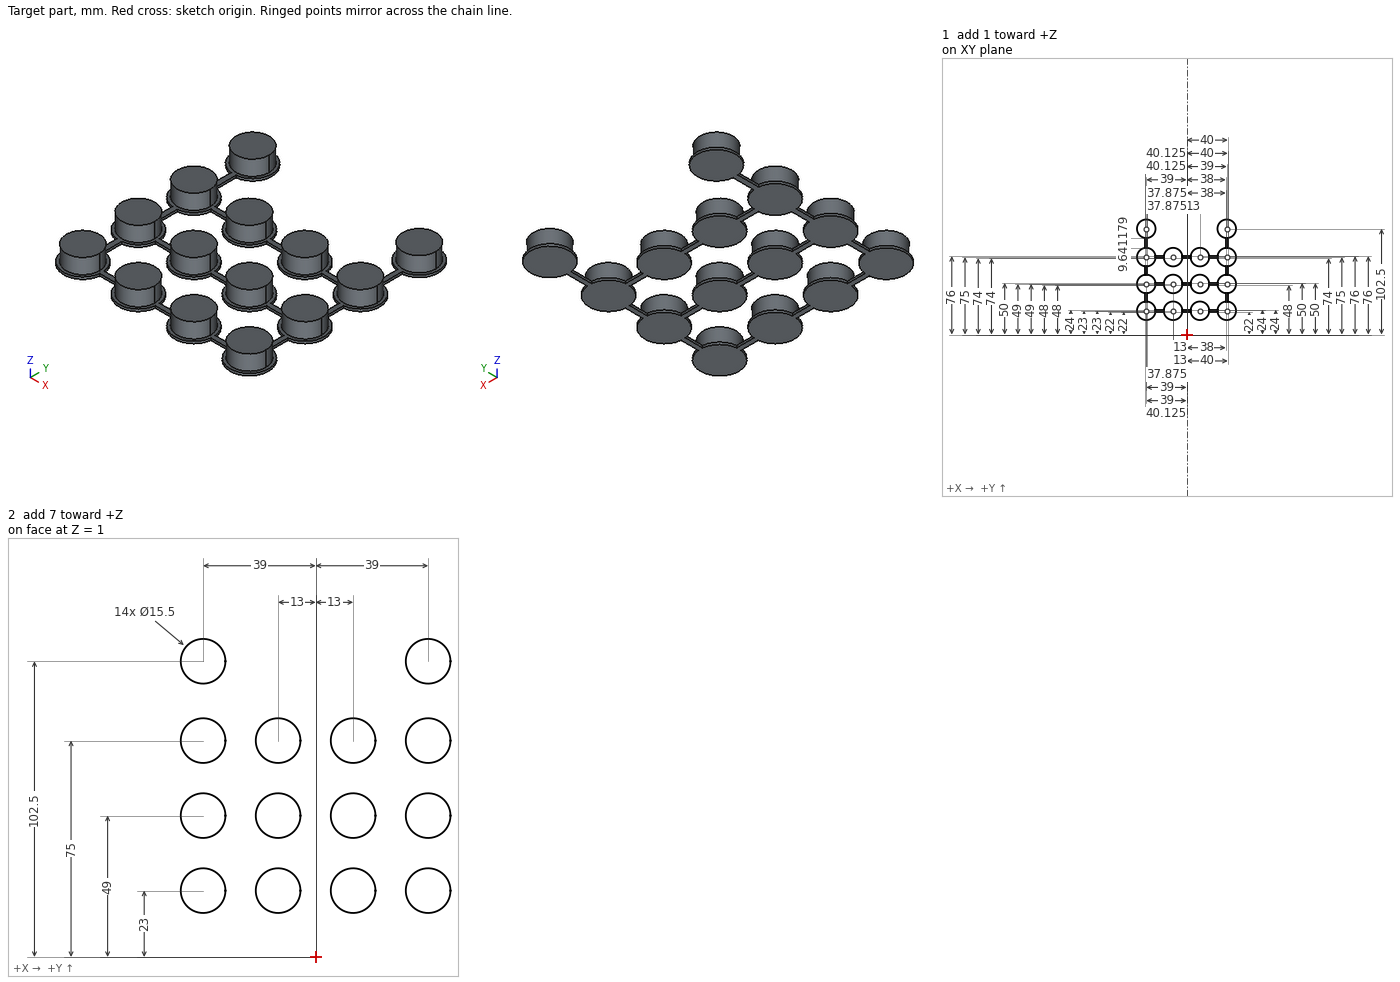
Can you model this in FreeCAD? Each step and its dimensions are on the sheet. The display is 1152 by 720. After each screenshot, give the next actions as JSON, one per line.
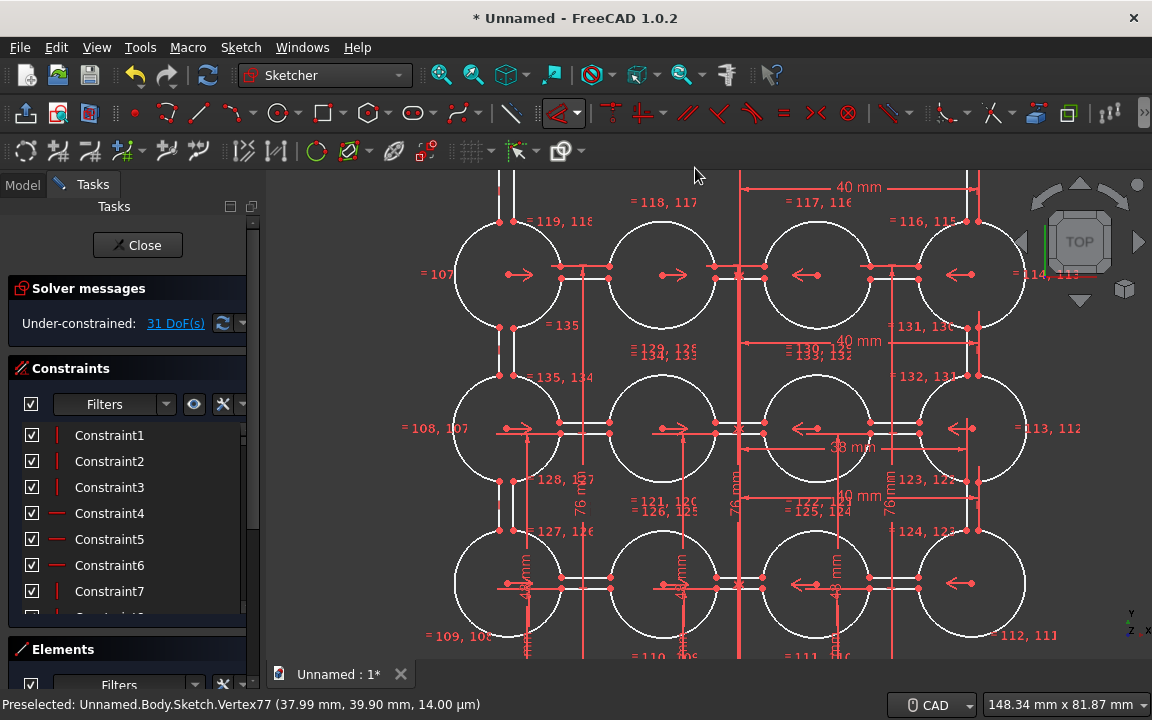
{"action": "left_click", "coordinate": [918, 578]}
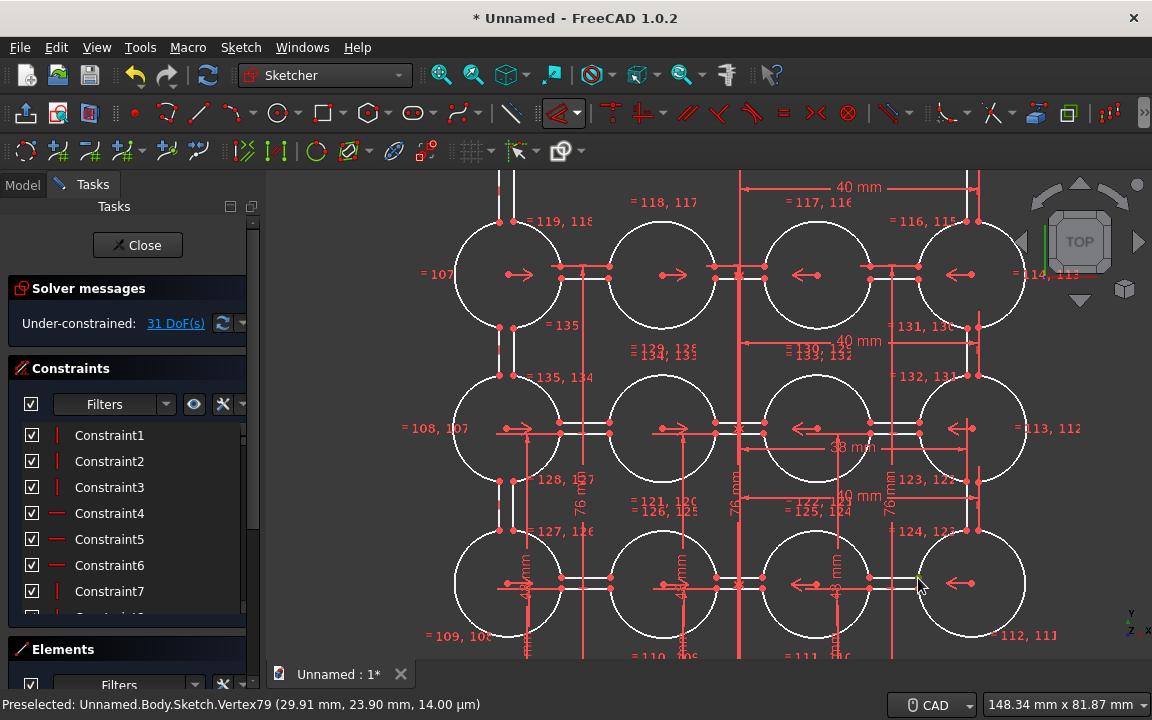
{"action": "key", "text": "i"}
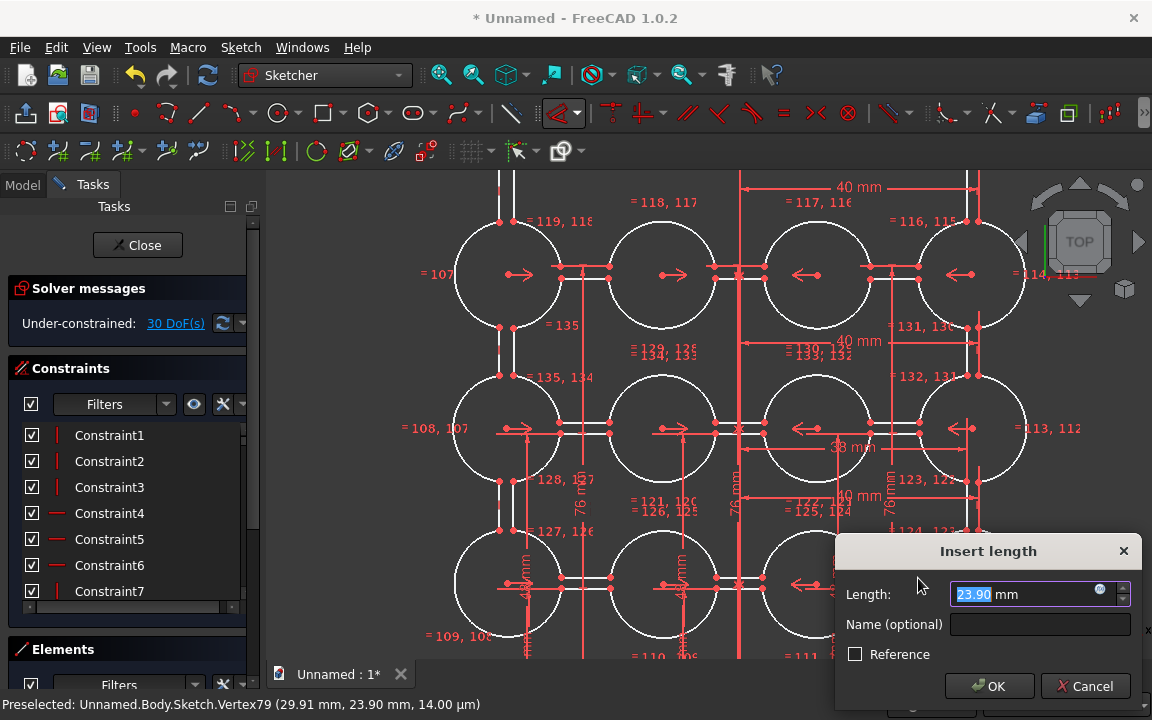
{"action": "type", "text": "24"}
{"action": "key", "text": "Return"}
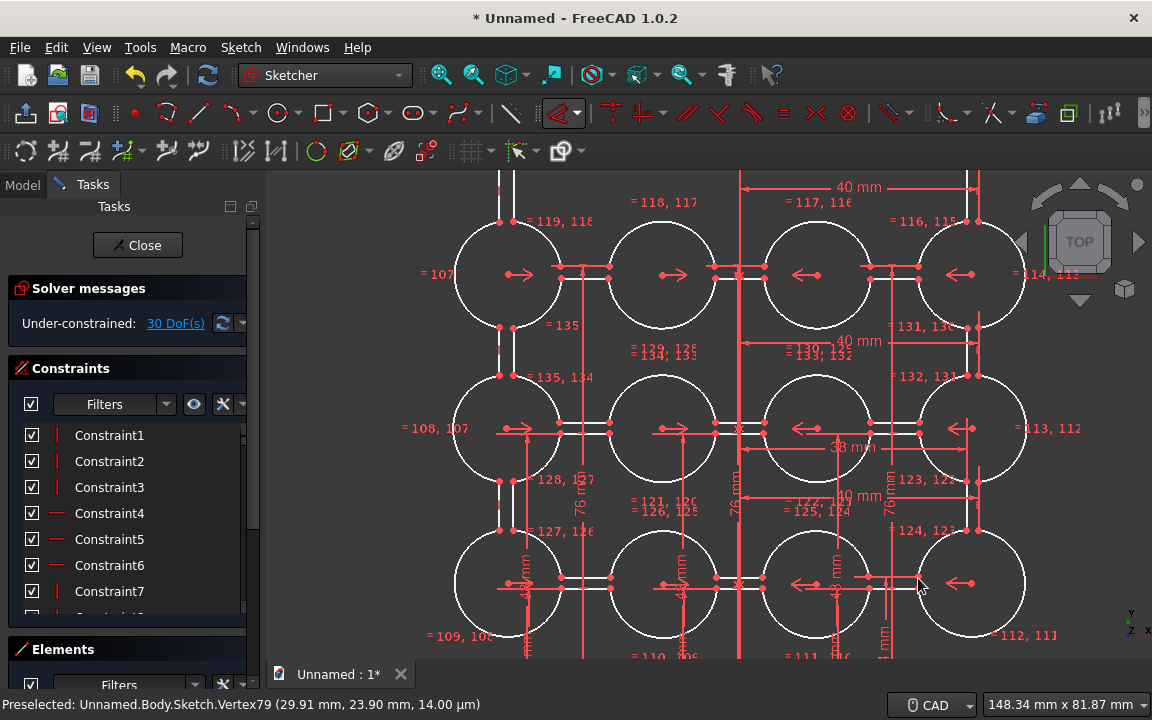
{"action": "left_click", "coordinate": [763, 578]}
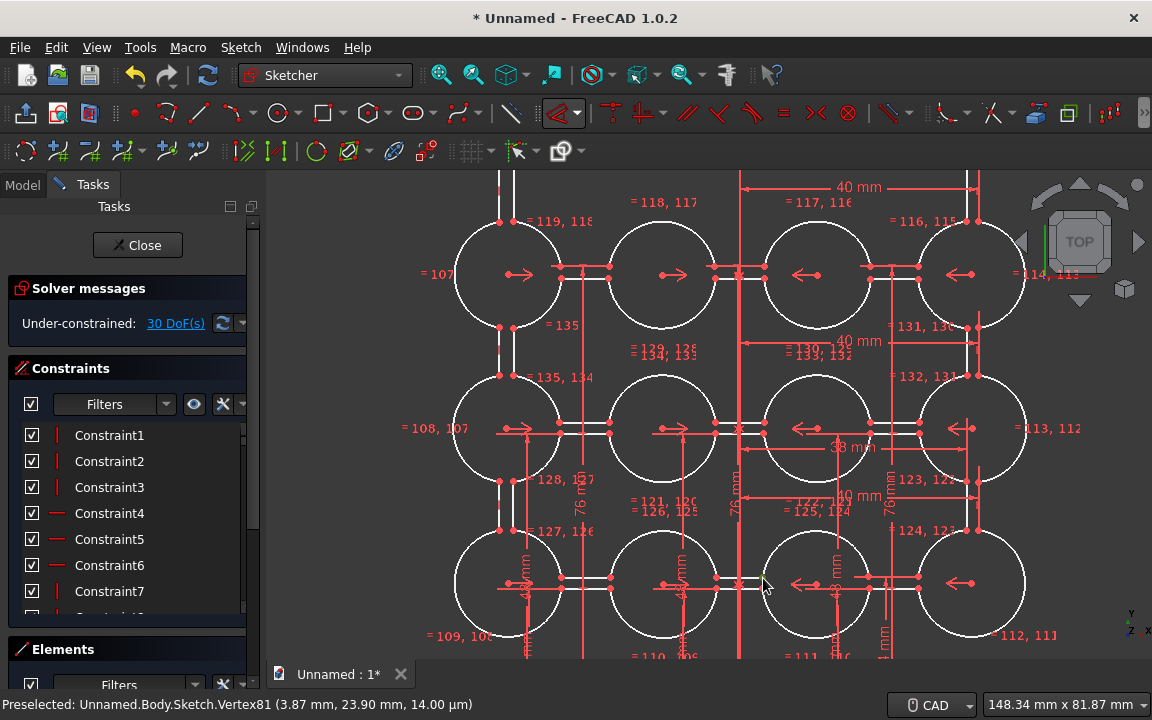
{"action": "left_click", "coordinate": [580, 114]}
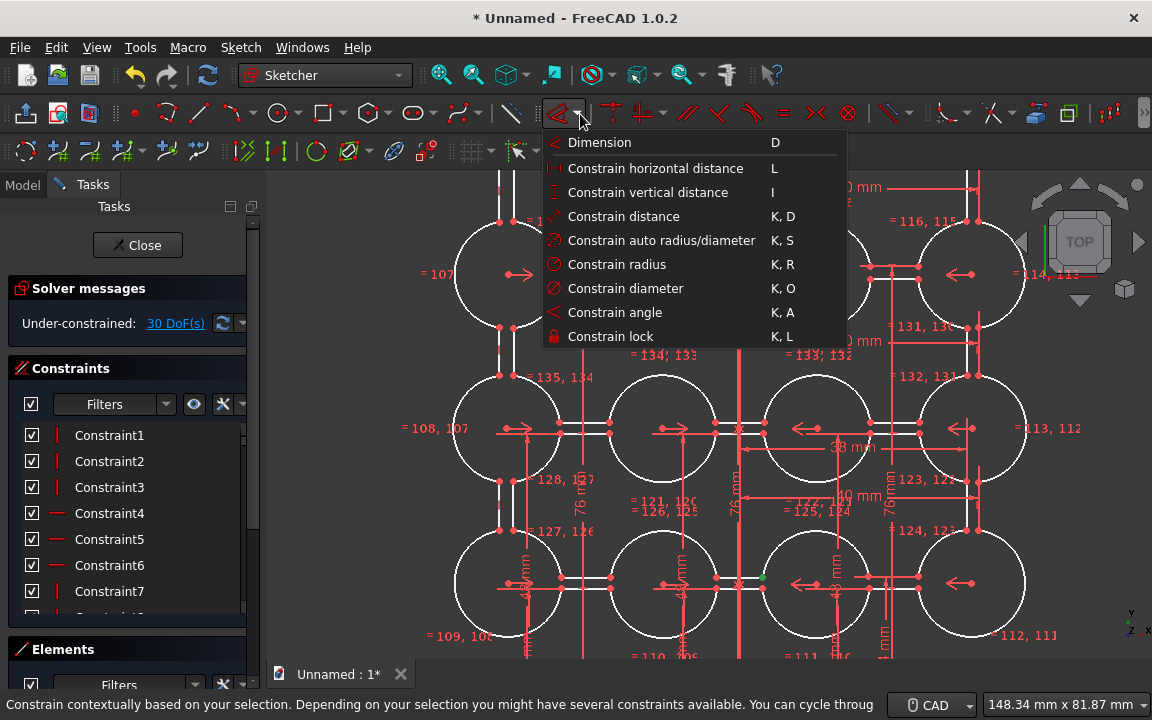
{"action": "left_click", "coordinate": [695, 192]}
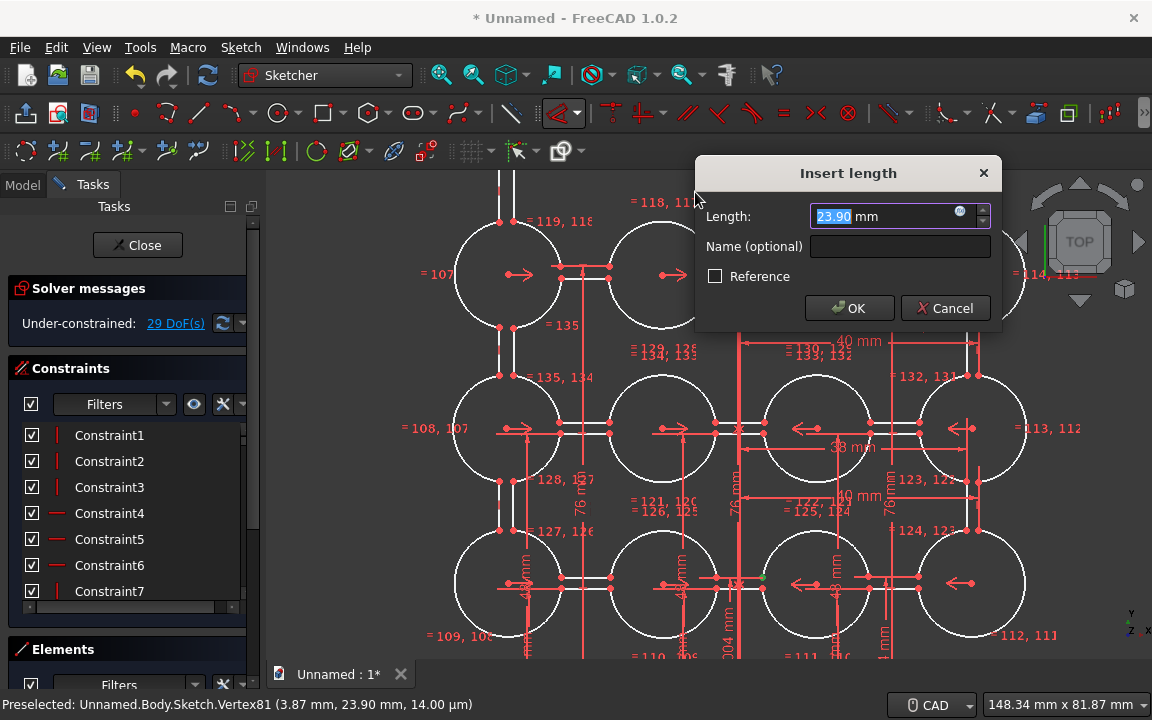
{"action": "type", "text": "24"}
{"action": "key", "text": "Return"}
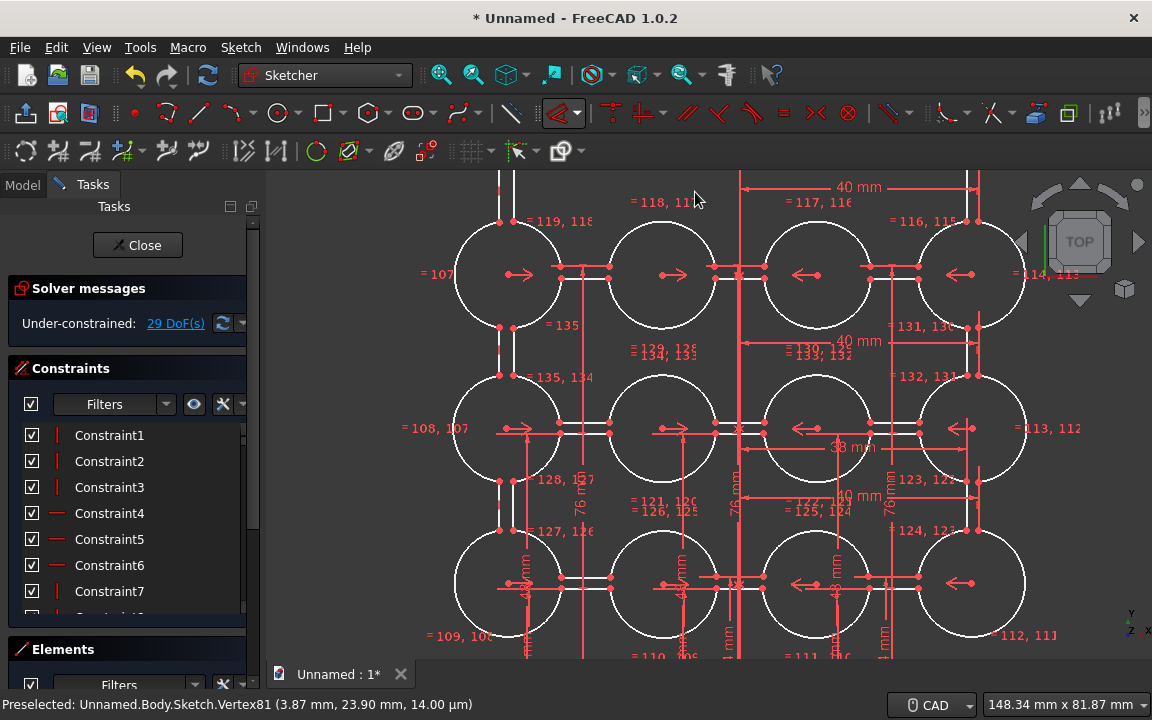
{"action": "left_click", "coordinate": [611, 578]}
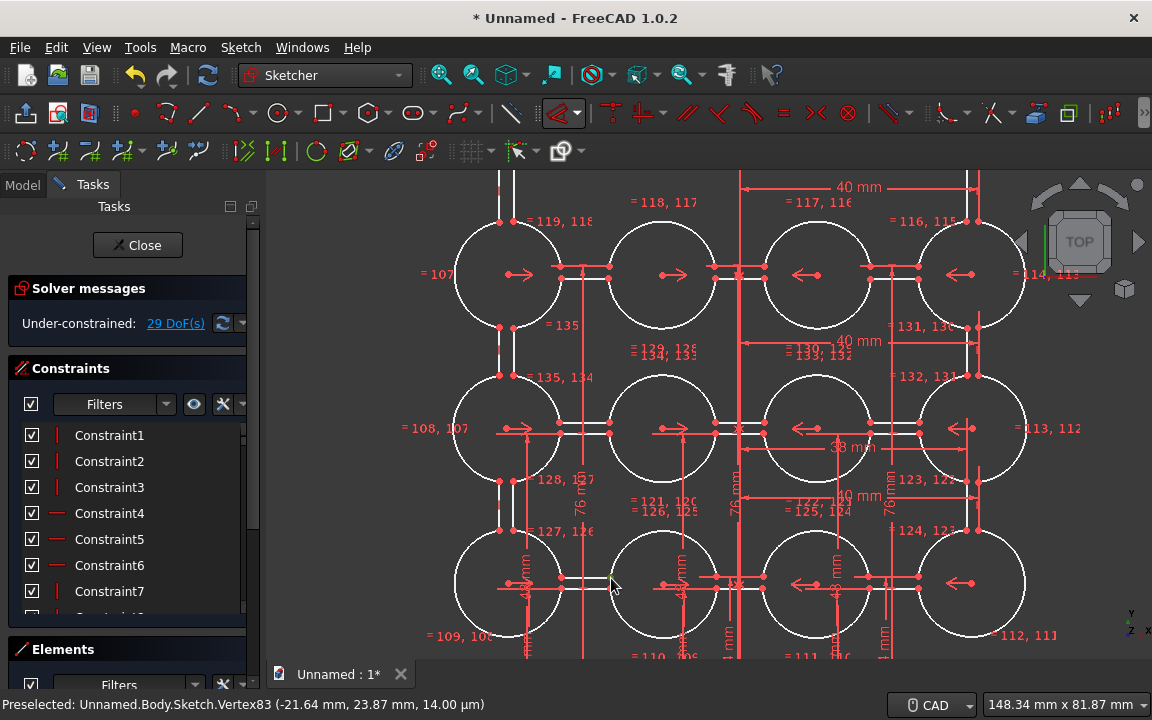
{"action": "left_click", "coordinate": [580, 114]}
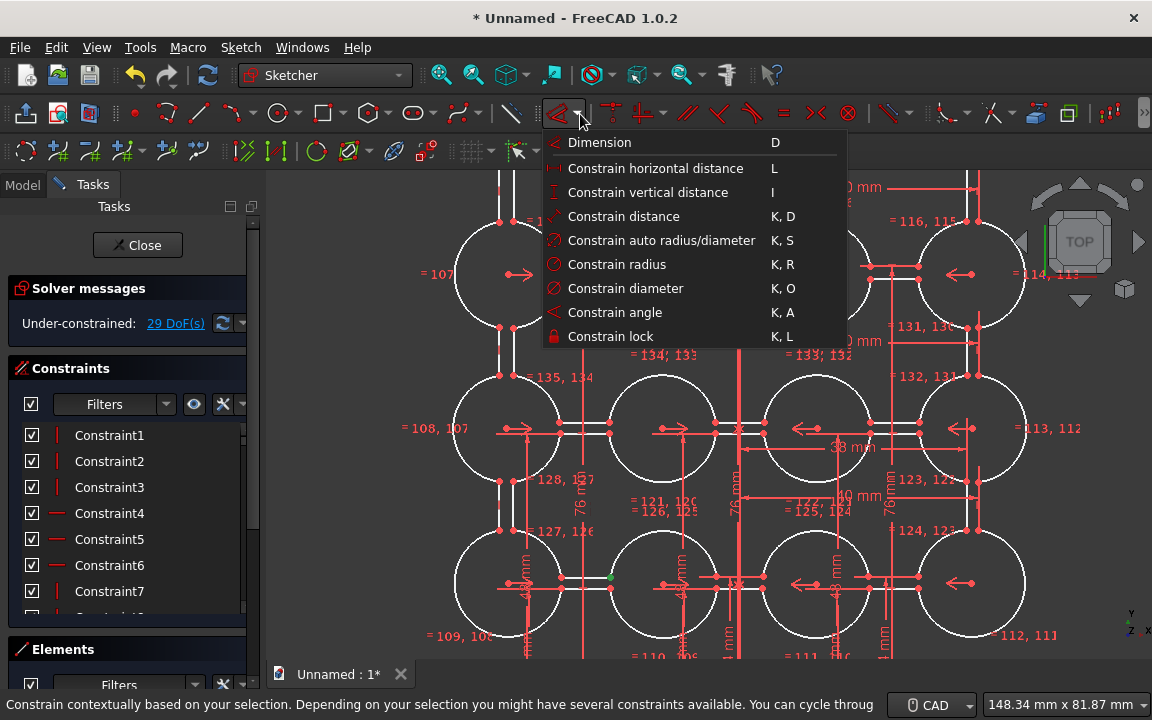
{"action": "left_click", "coordinate": [695, 192]}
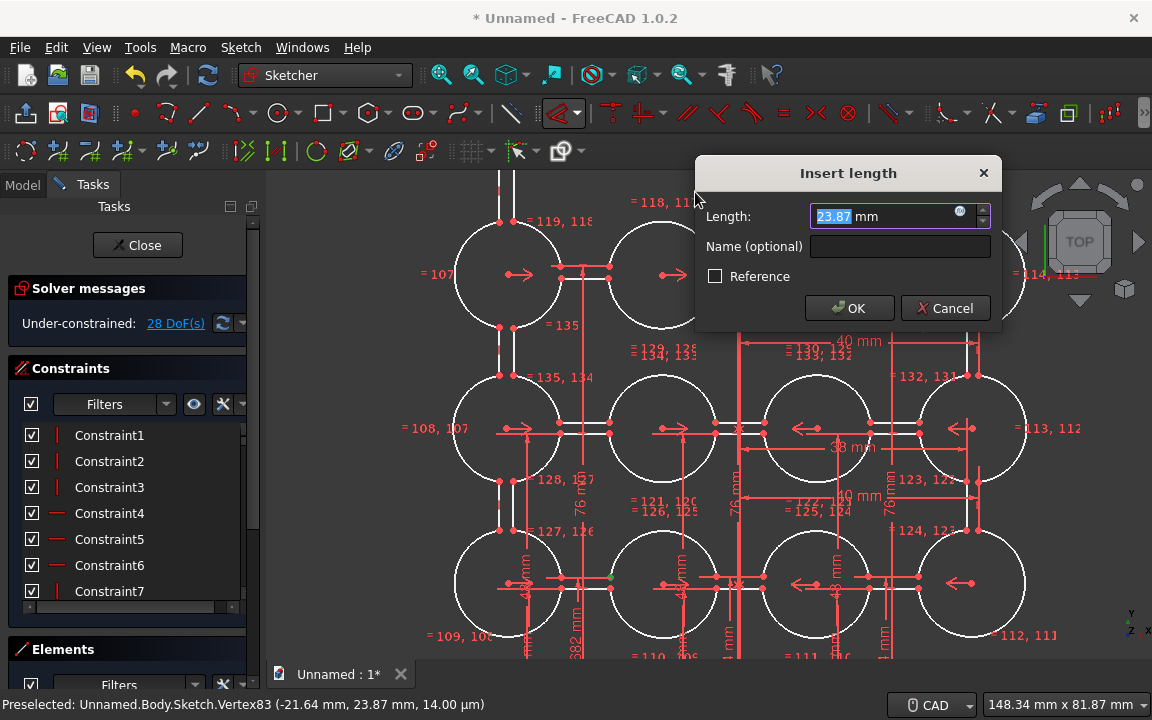
{"action": "type", "text": "24"}
{"action": "key", "text": "Return"}